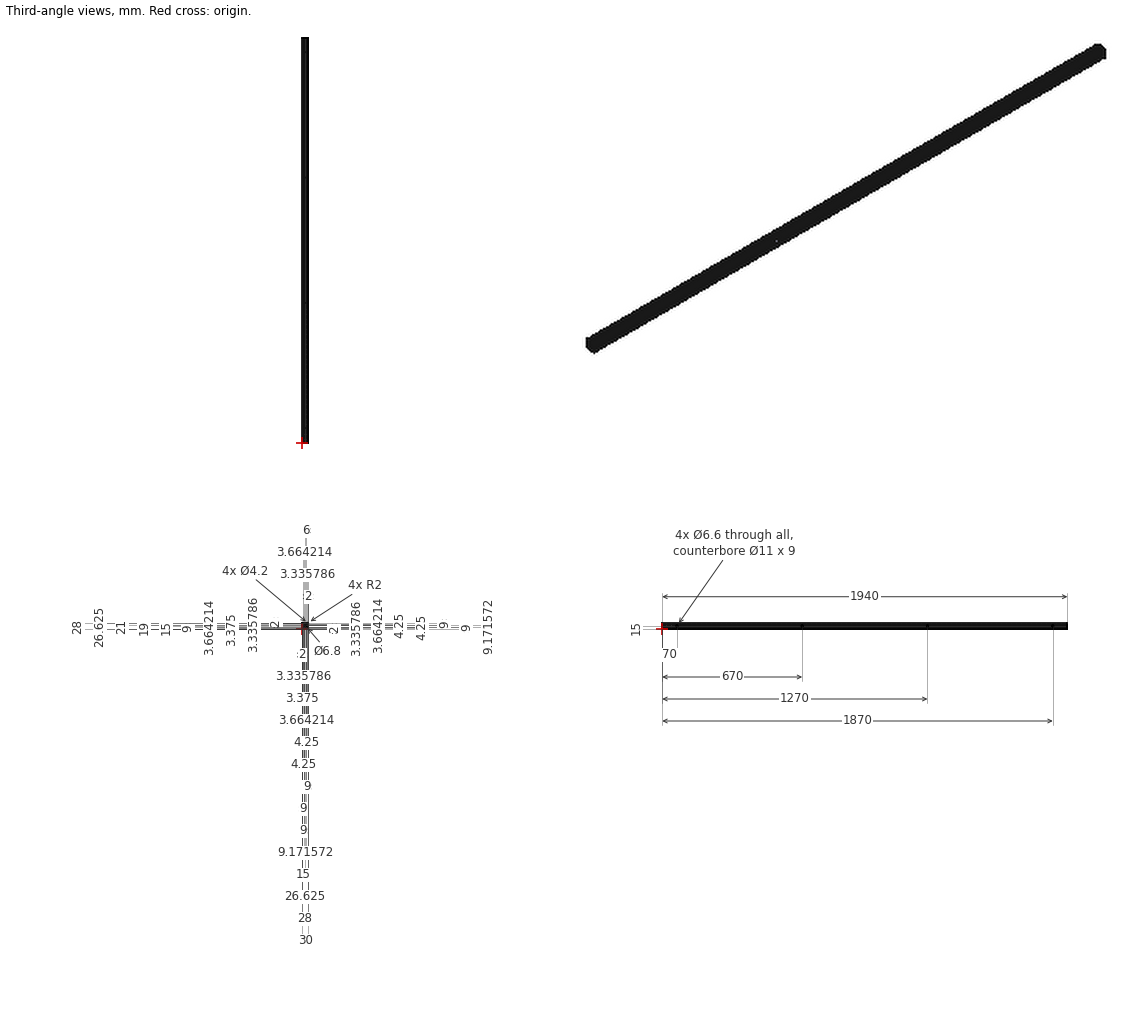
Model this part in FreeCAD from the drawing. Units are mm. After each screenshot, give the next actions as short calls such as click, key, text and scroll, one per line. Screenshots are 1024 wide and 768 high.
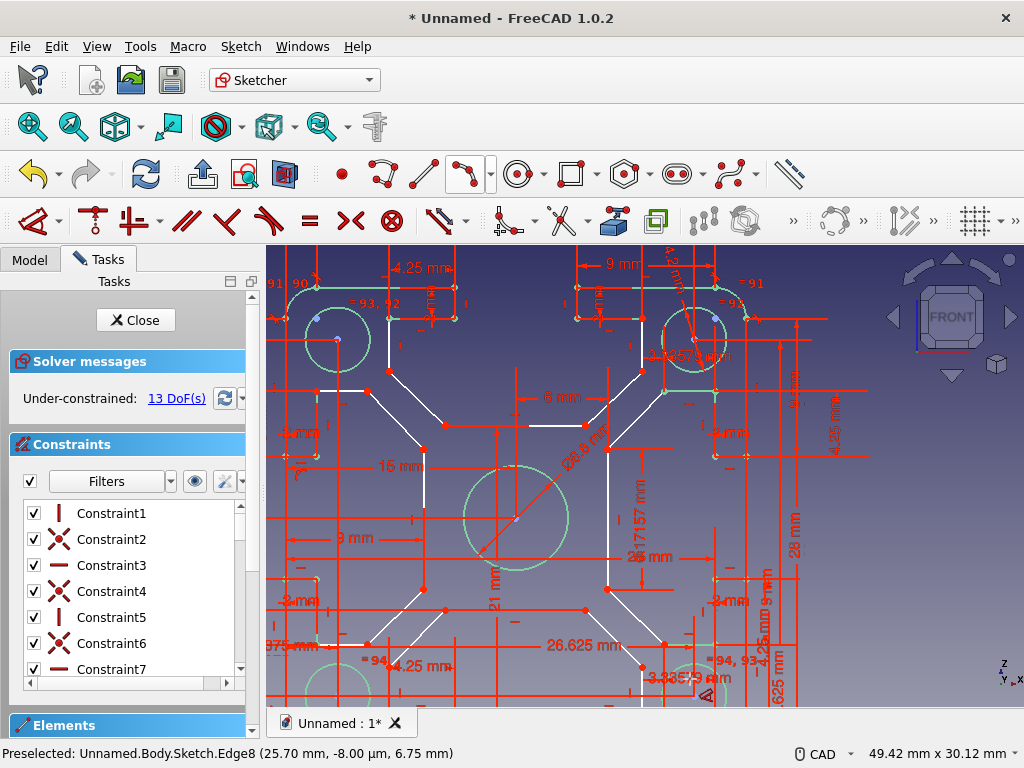
scroll(642, 677, up, 2)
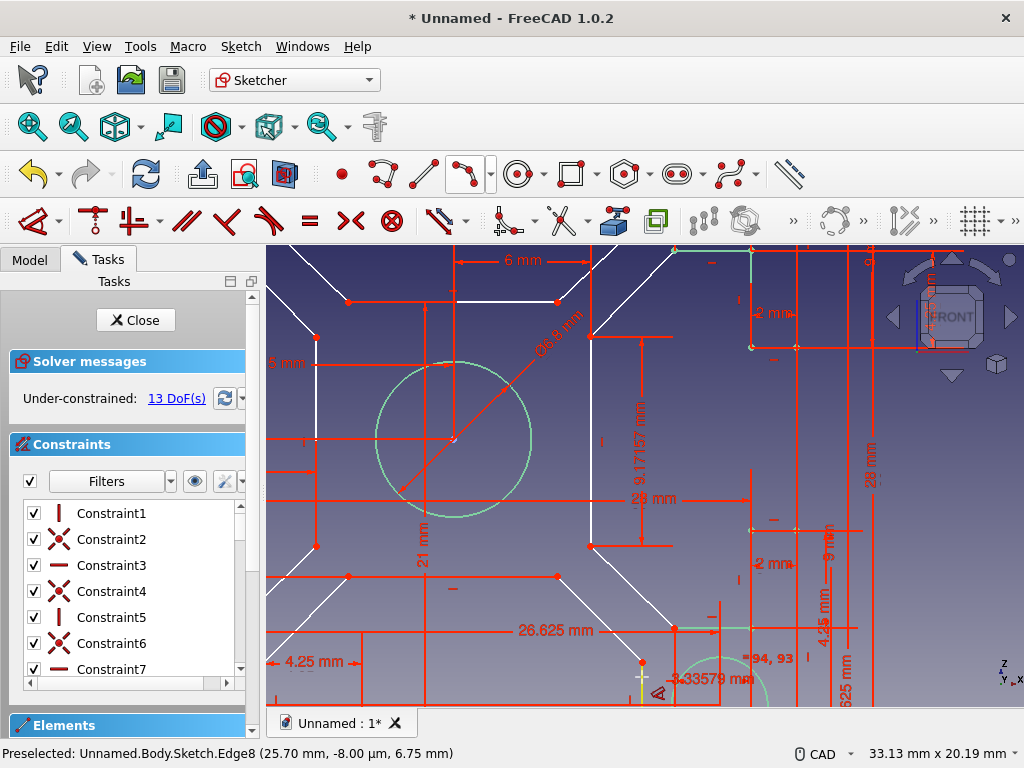
click(642, 677)
click(608, 671)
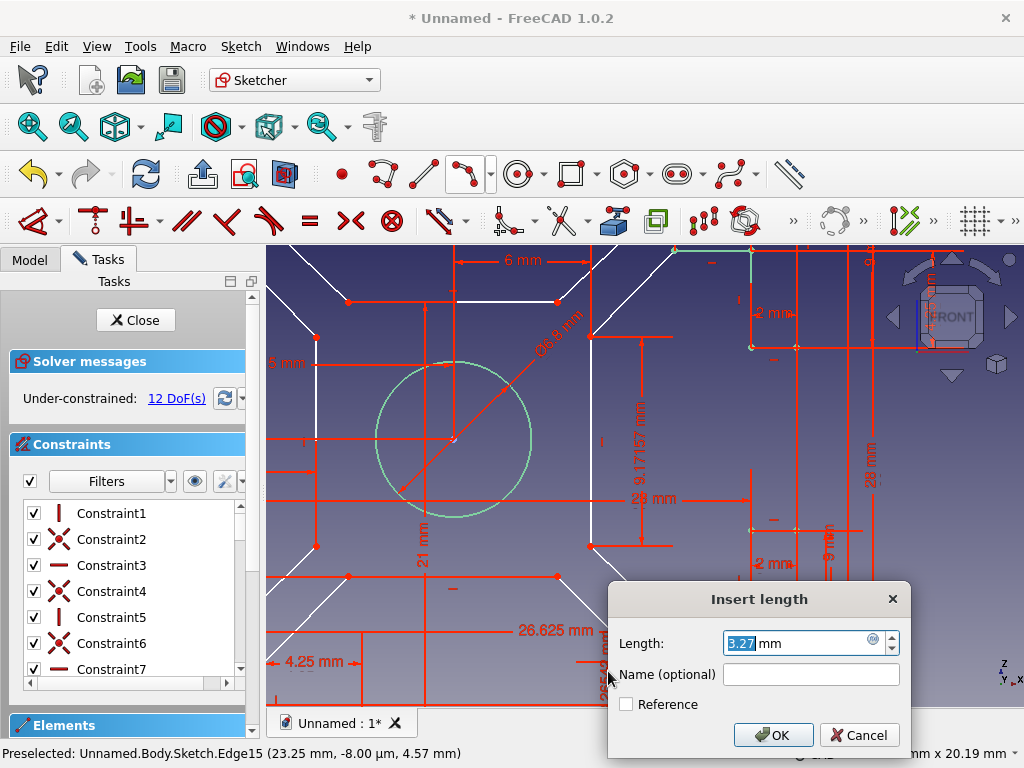
text(3.335786)
key(Return)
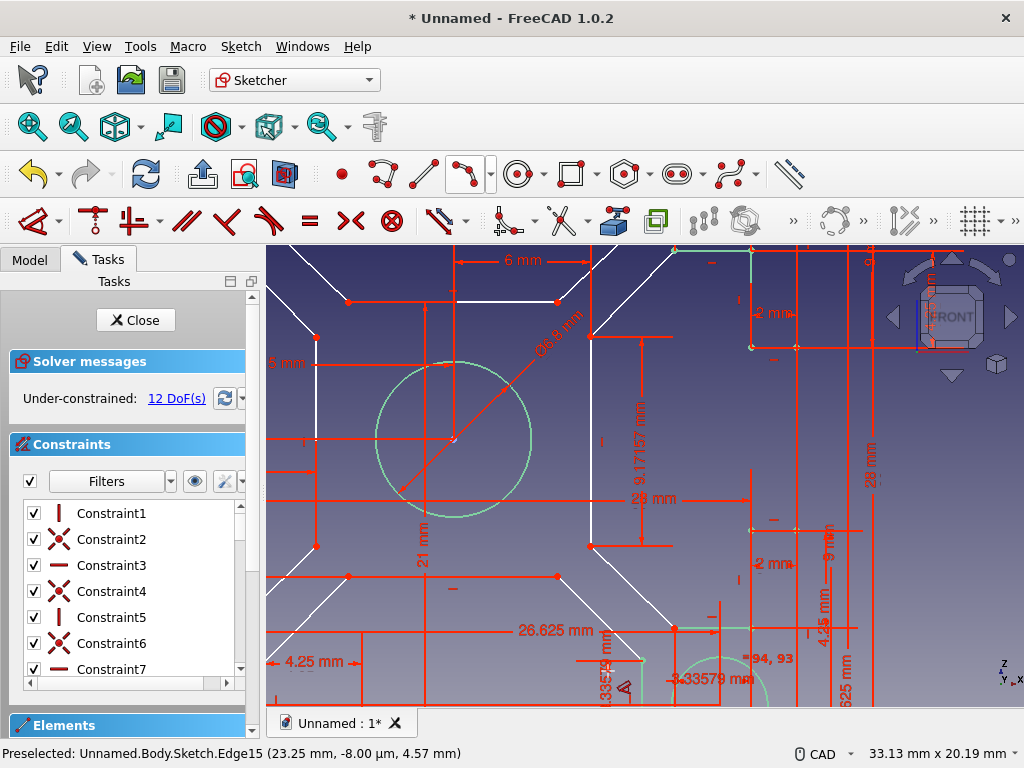
click(495, 577)
click(453, 611)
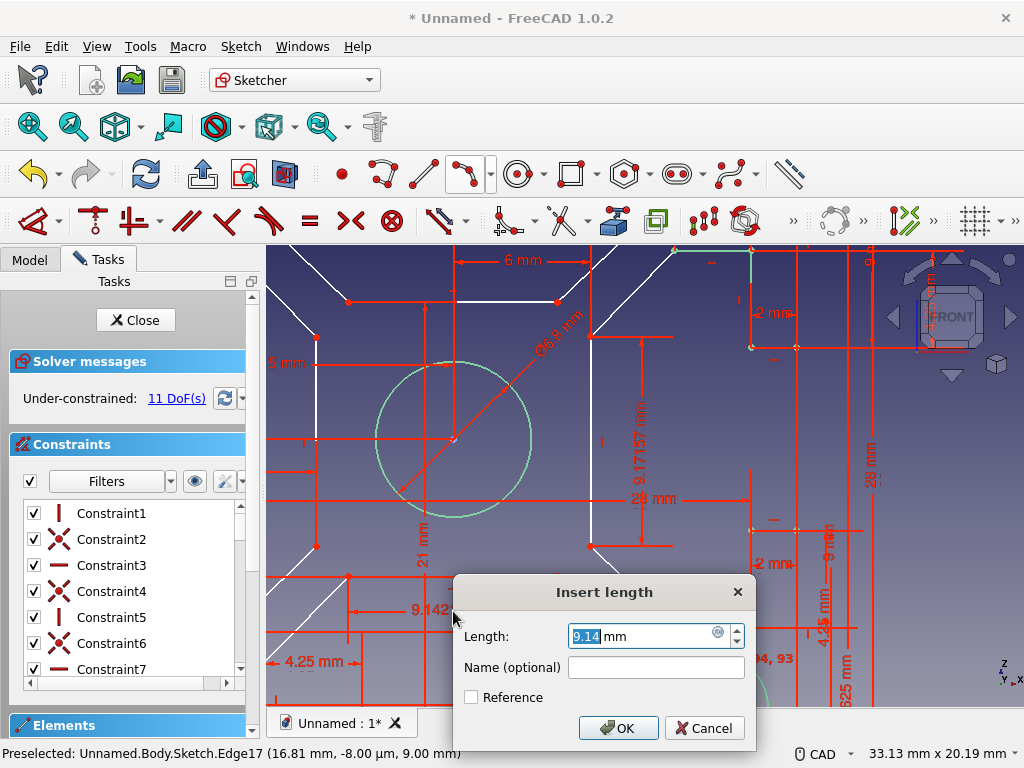
text(9.171572)
key(Return)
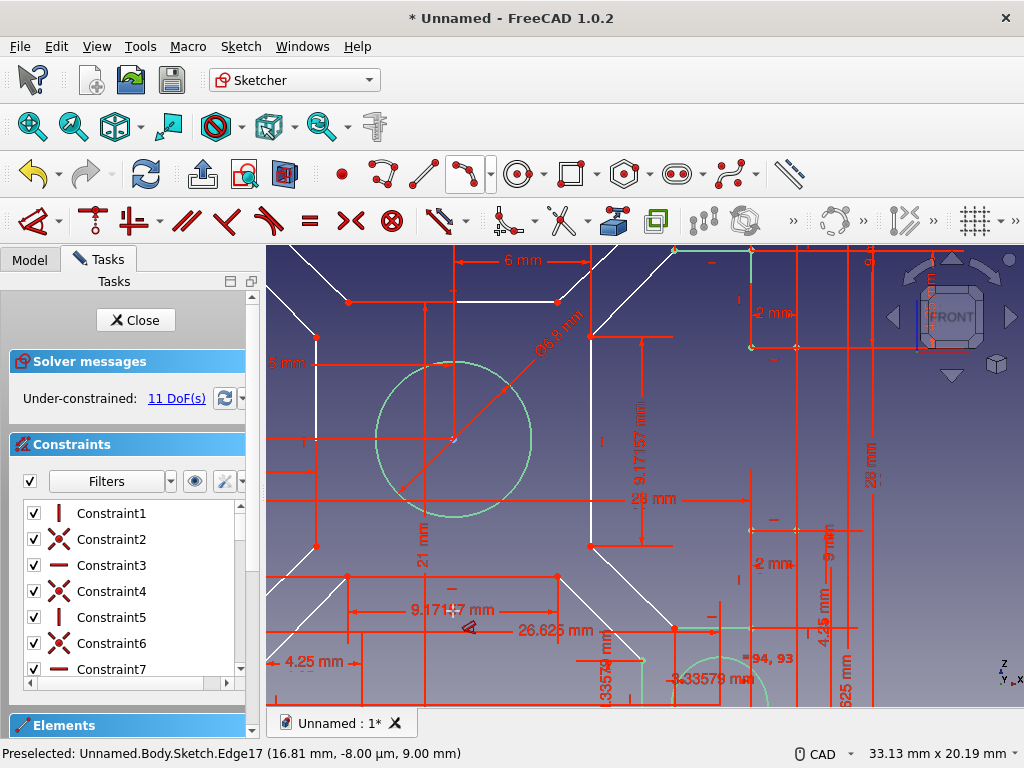
scroll(677, 506, down, 4)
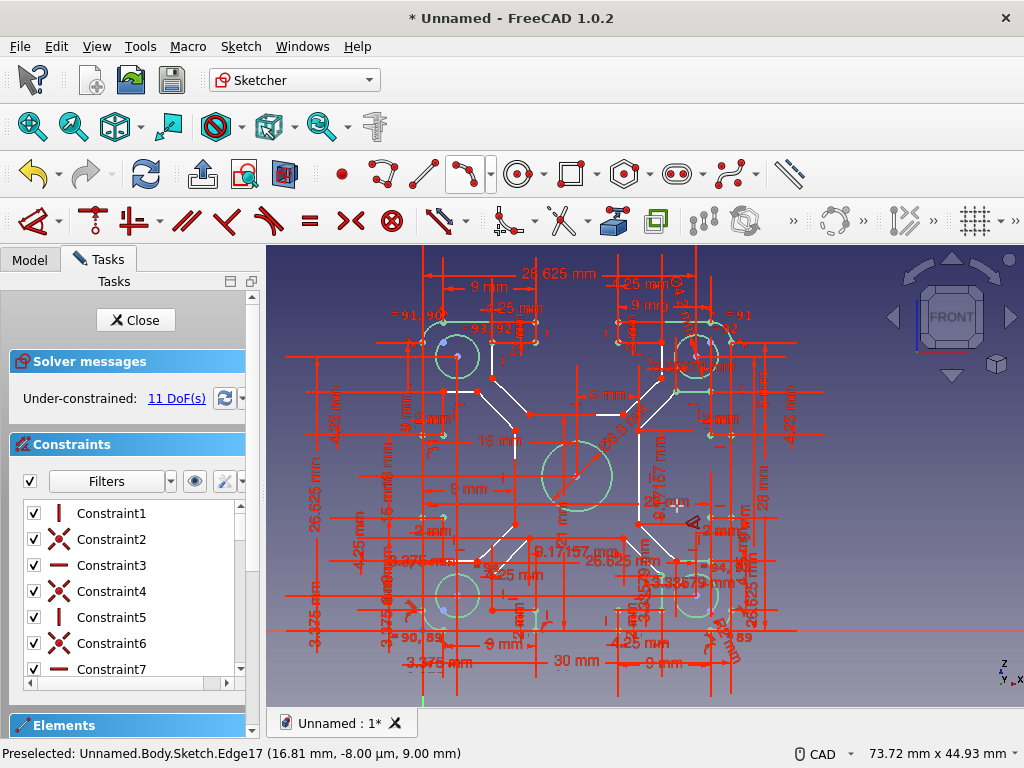
scroll(492, 587, up, 2)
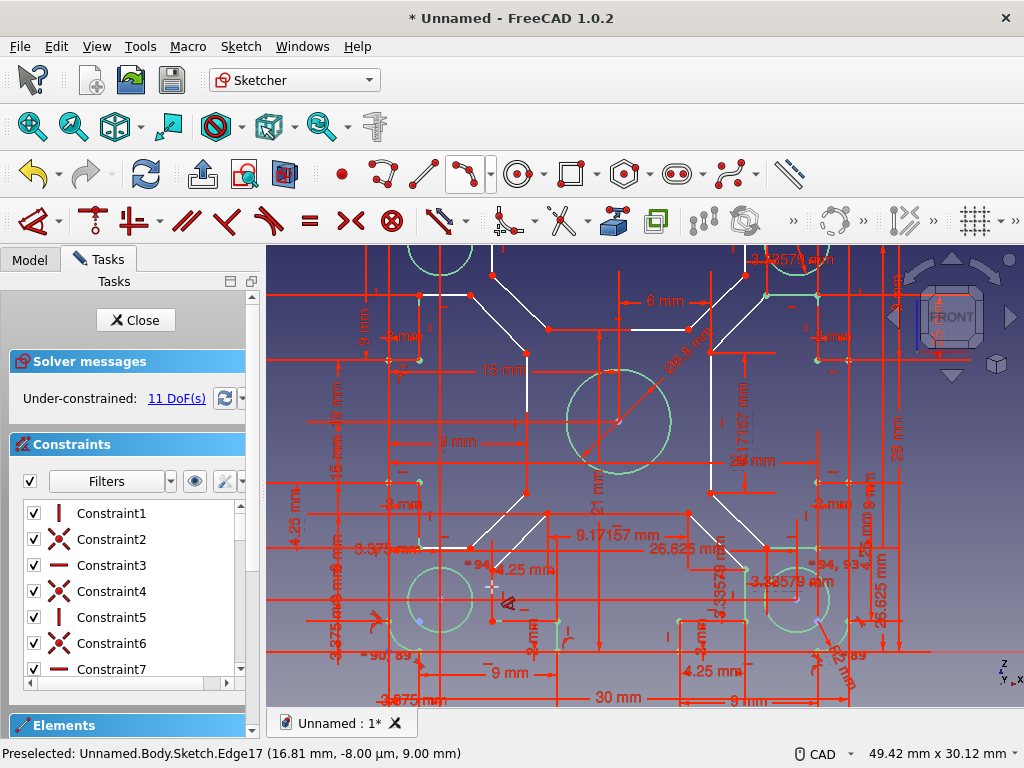
click(492, 586)
click(458, 596)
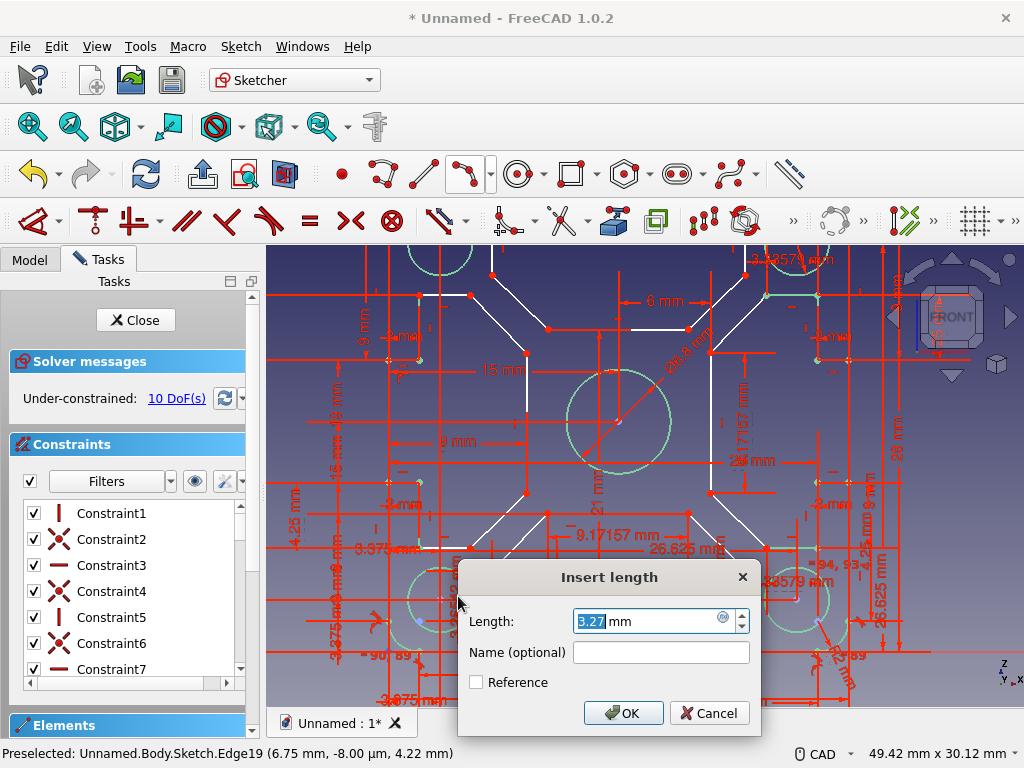
text(3.335786)
key(Return)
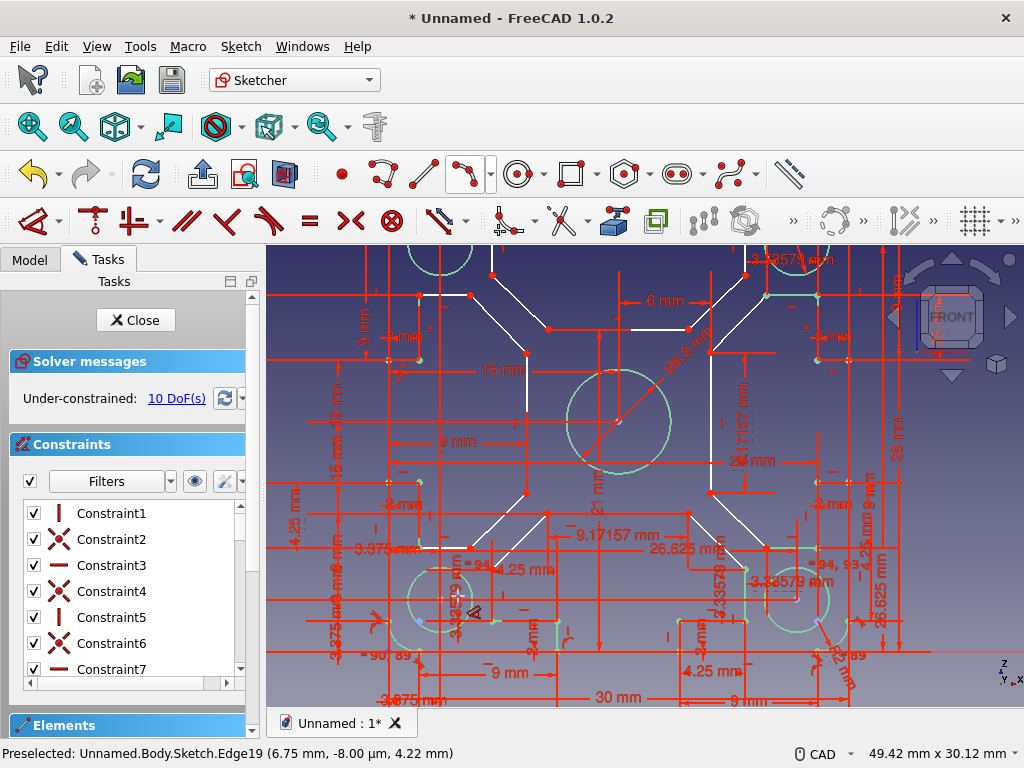
click(435, 548)
click(445, 466)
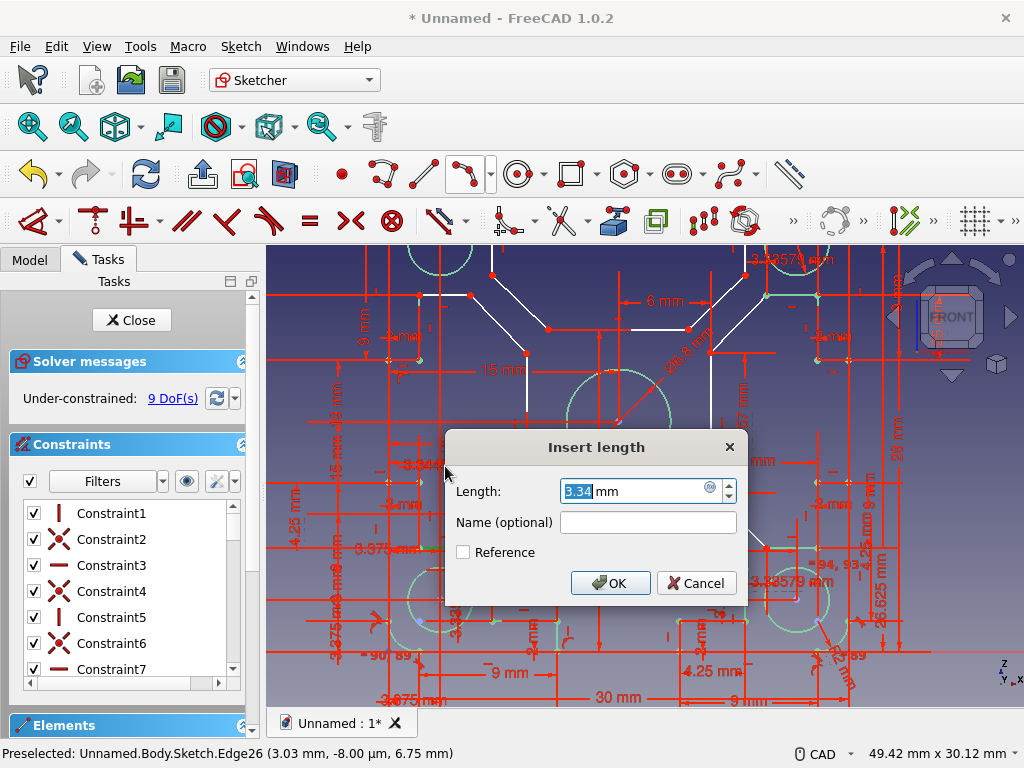
text(3.335786)
key(Return)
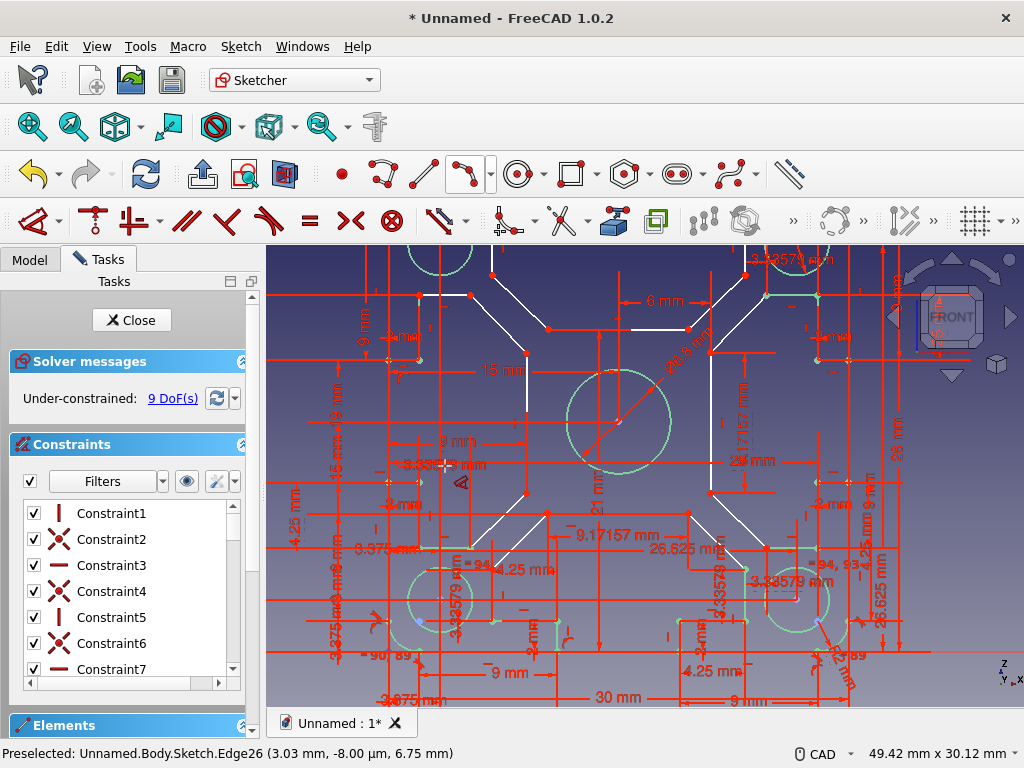
click(527, 451)
click(561, 455)